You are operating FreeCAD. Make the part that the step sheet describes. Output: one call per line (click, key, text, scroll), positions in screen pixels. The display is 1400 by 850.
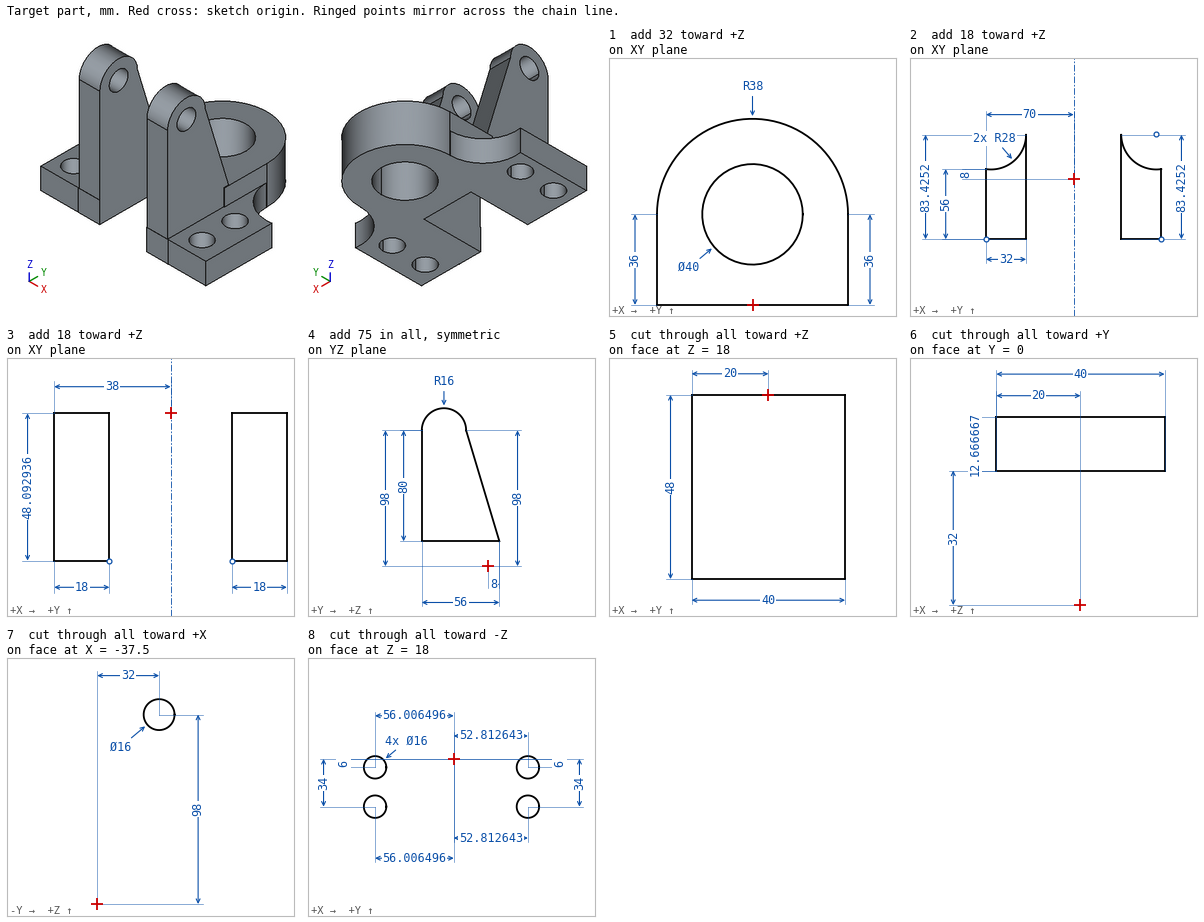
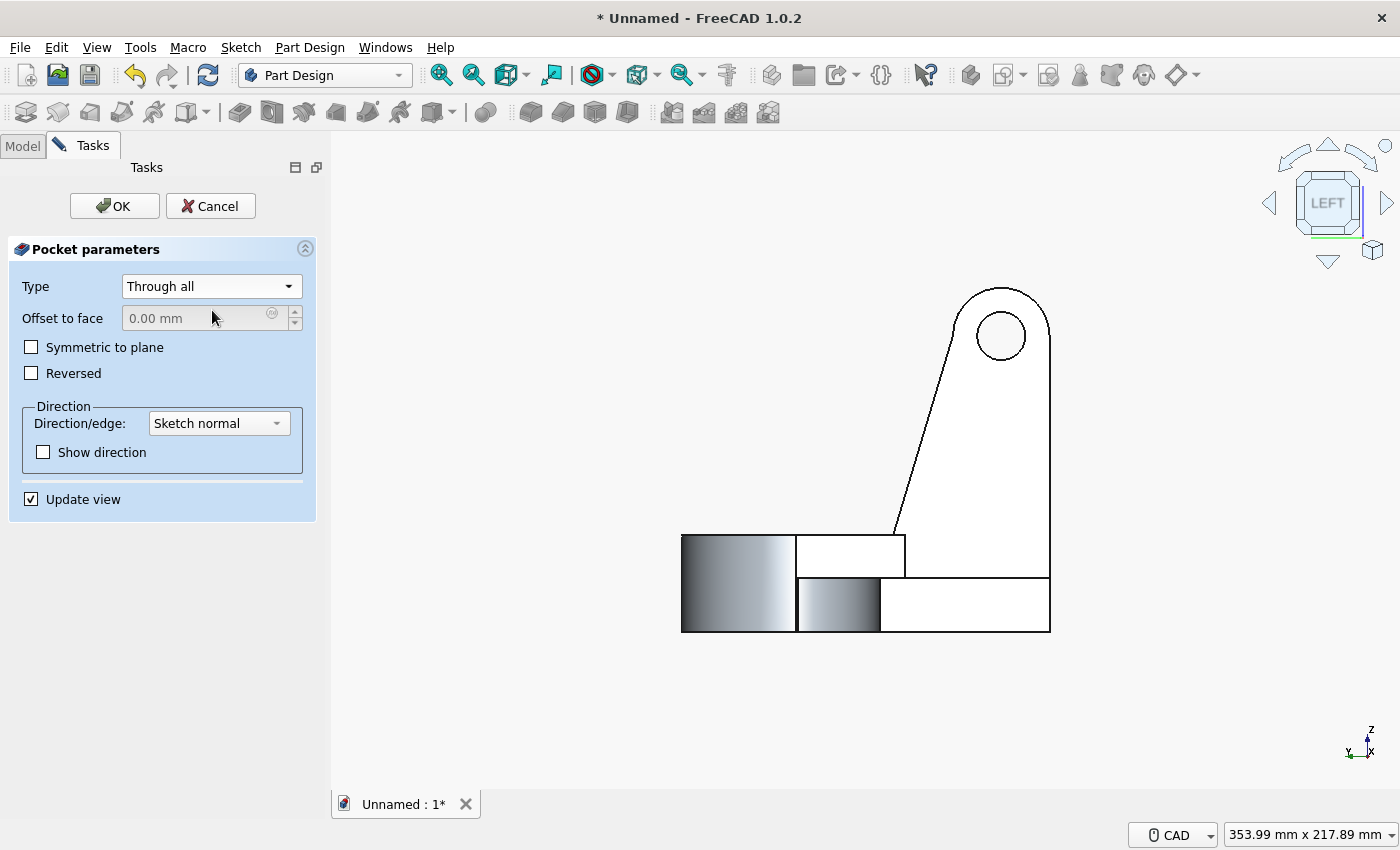
click(115, 206)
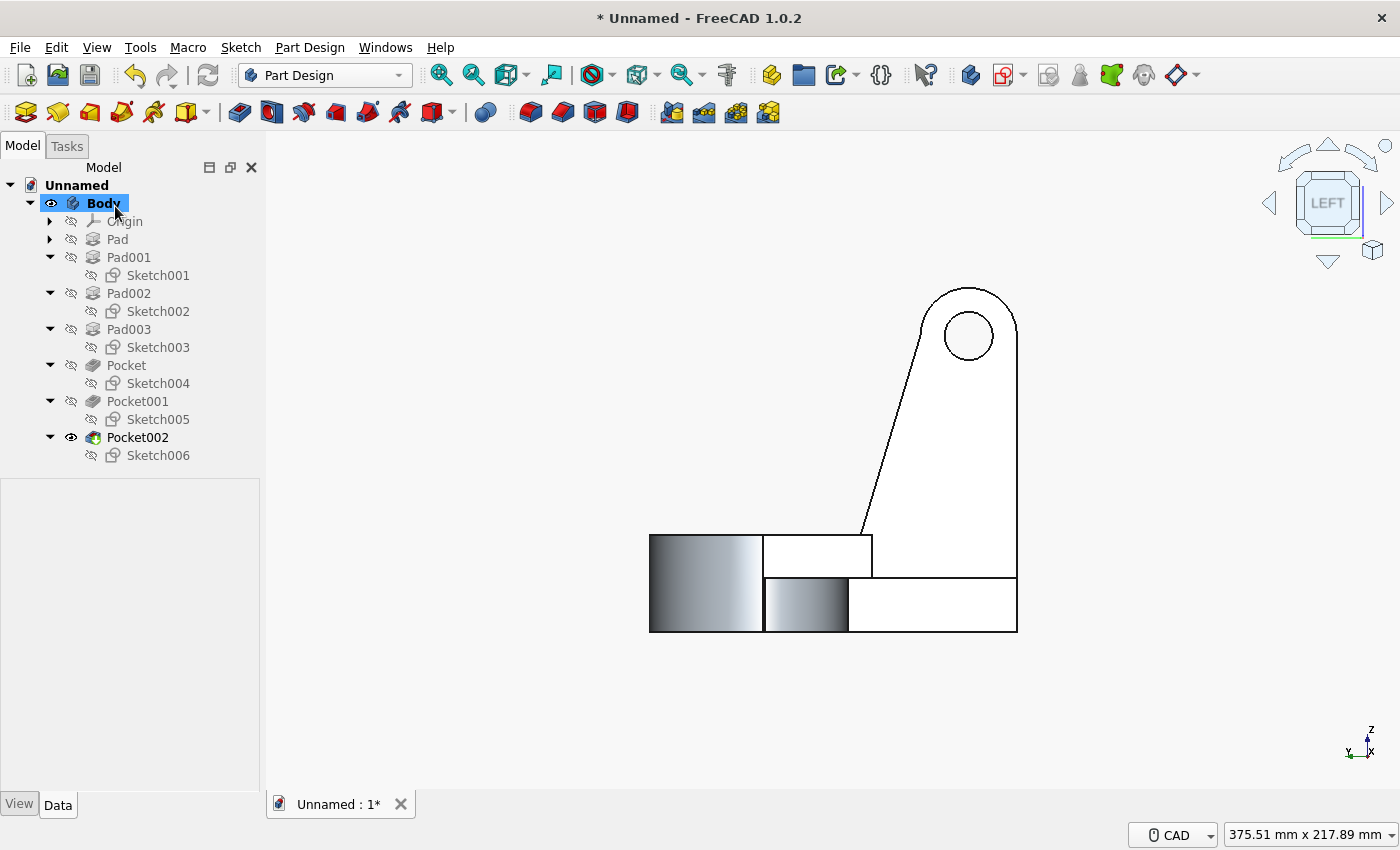
key(0)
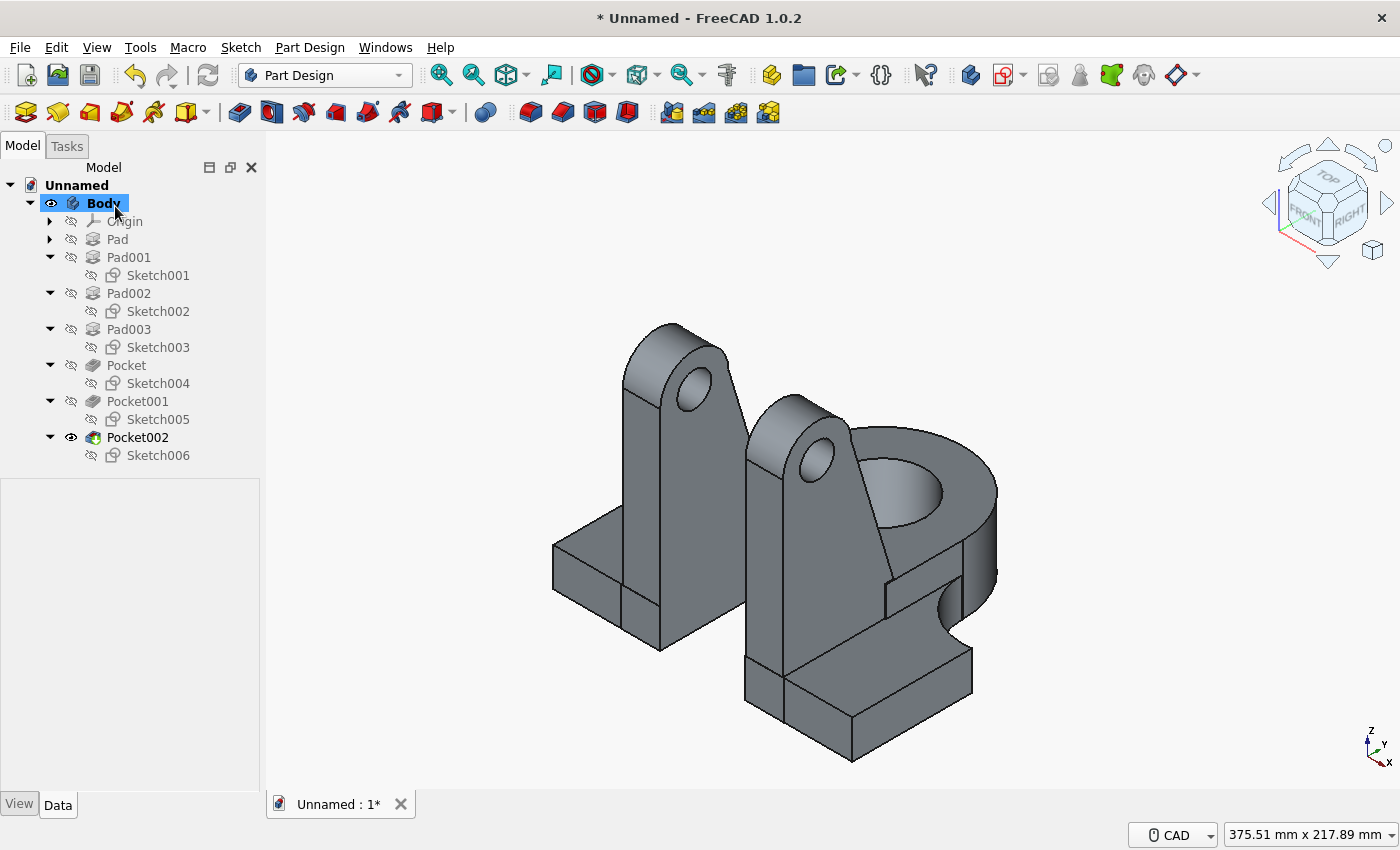
click(614, 535)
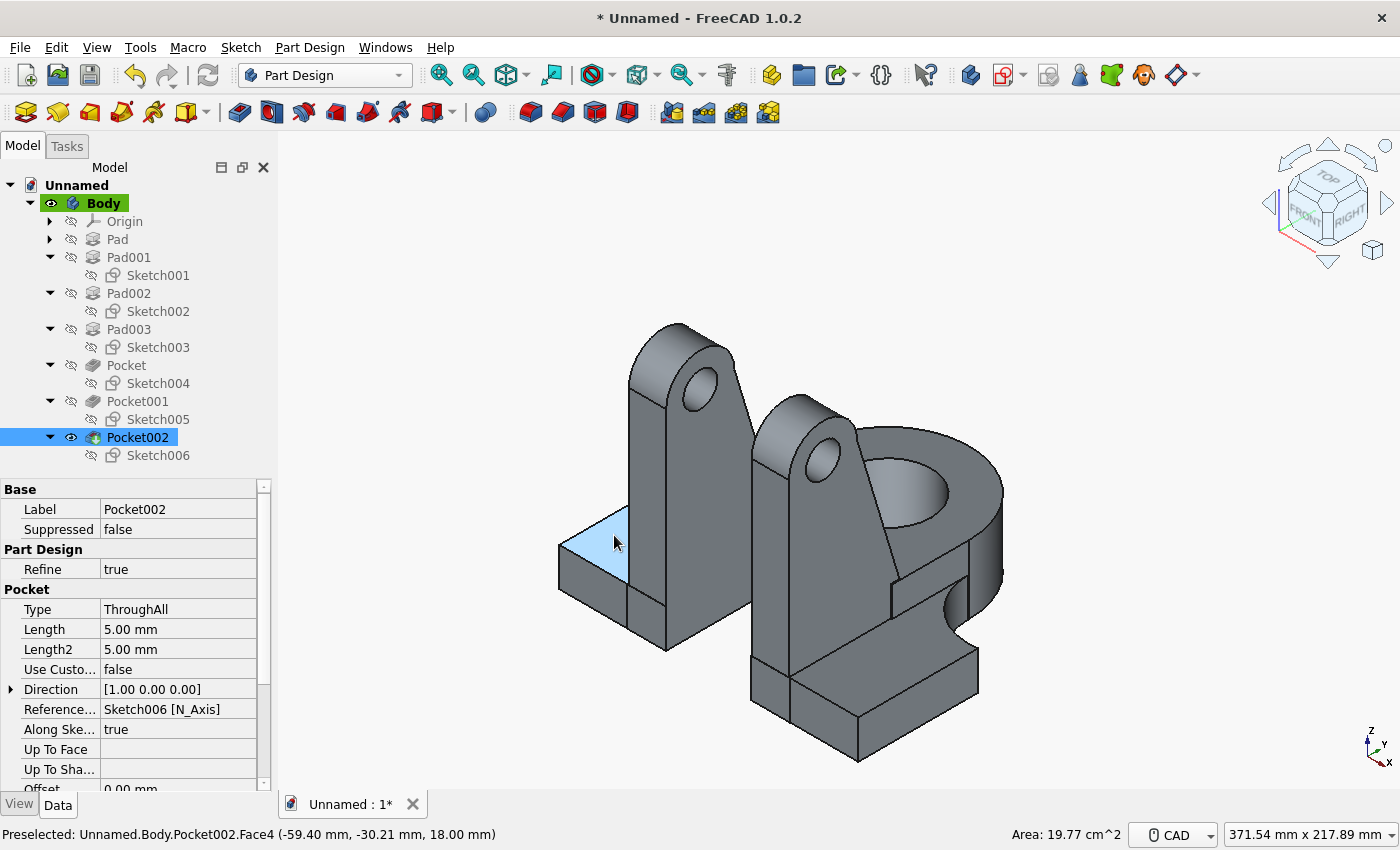
click(1004, 76)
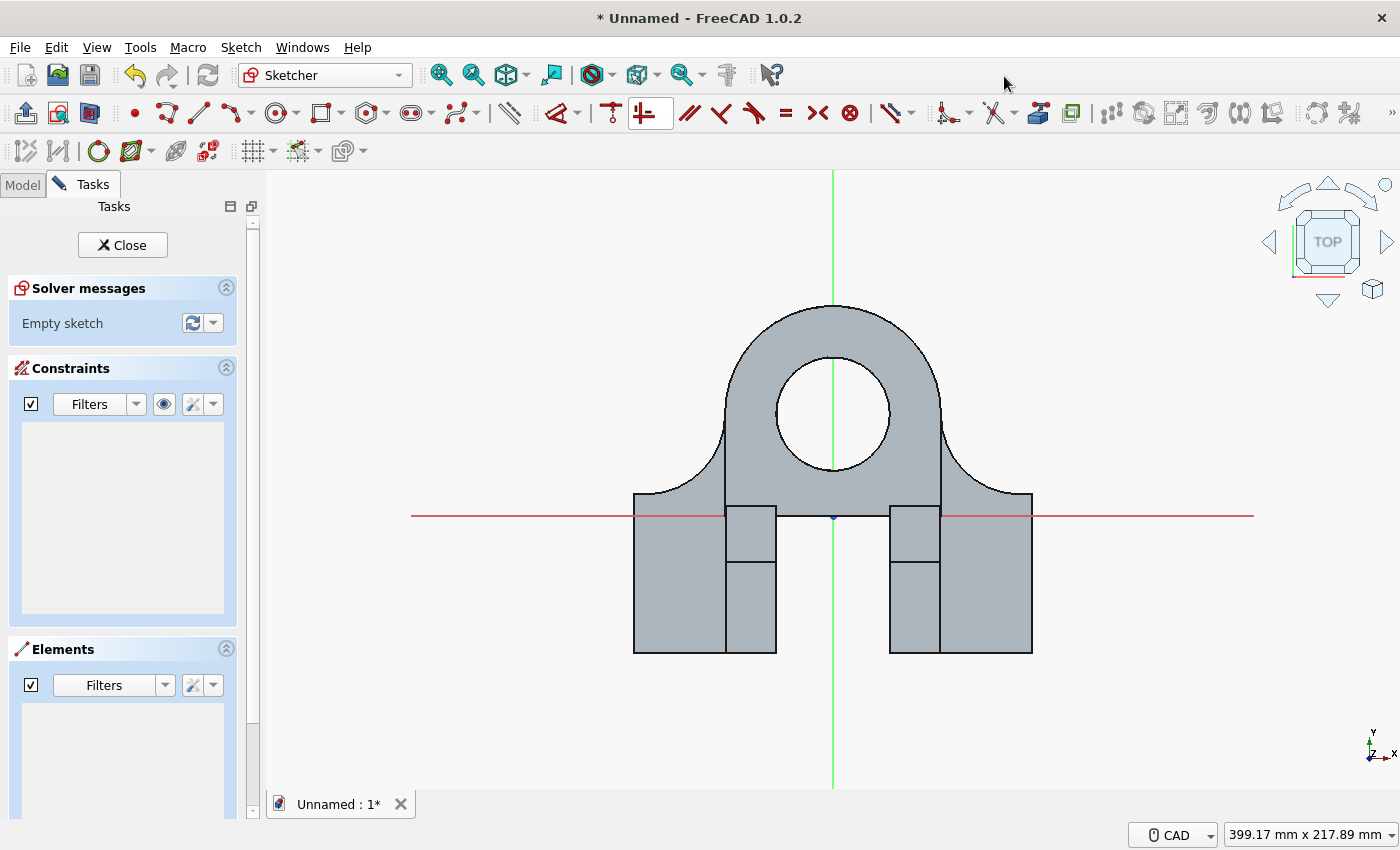
click(90, 114)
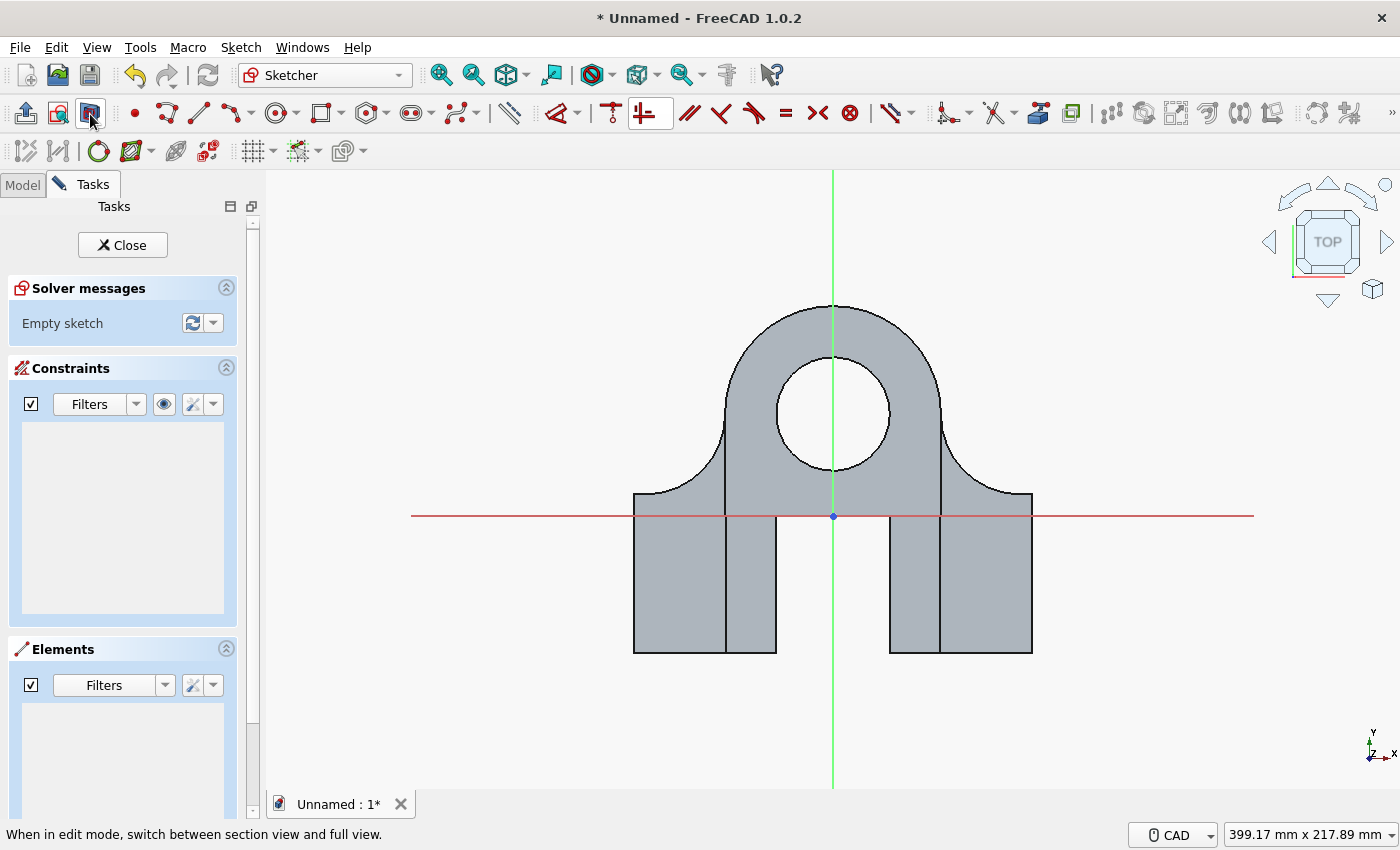
scroll(906, 687, up, 3)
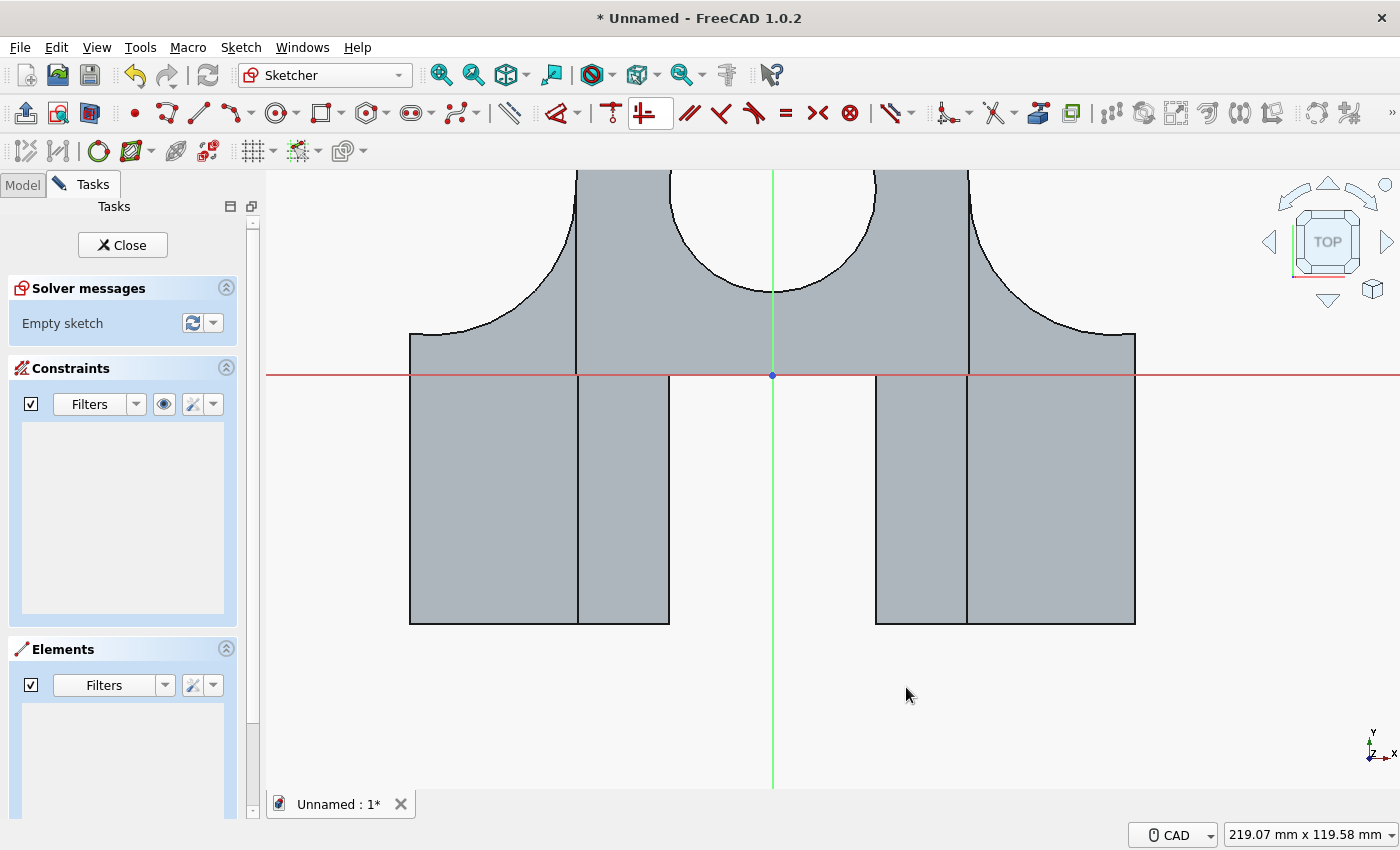
click(276, 114)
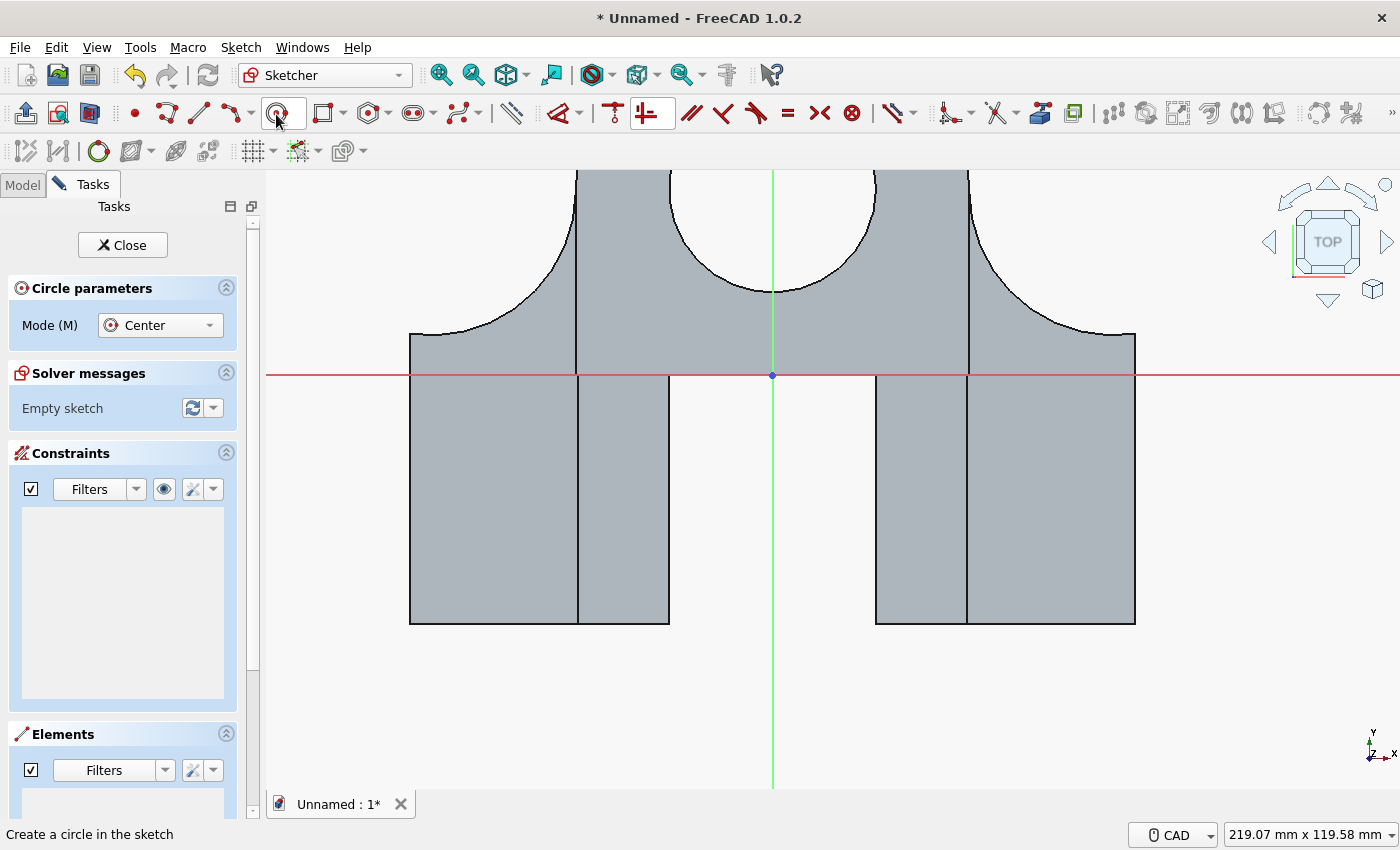
click(483, 406)
click(512, 436)